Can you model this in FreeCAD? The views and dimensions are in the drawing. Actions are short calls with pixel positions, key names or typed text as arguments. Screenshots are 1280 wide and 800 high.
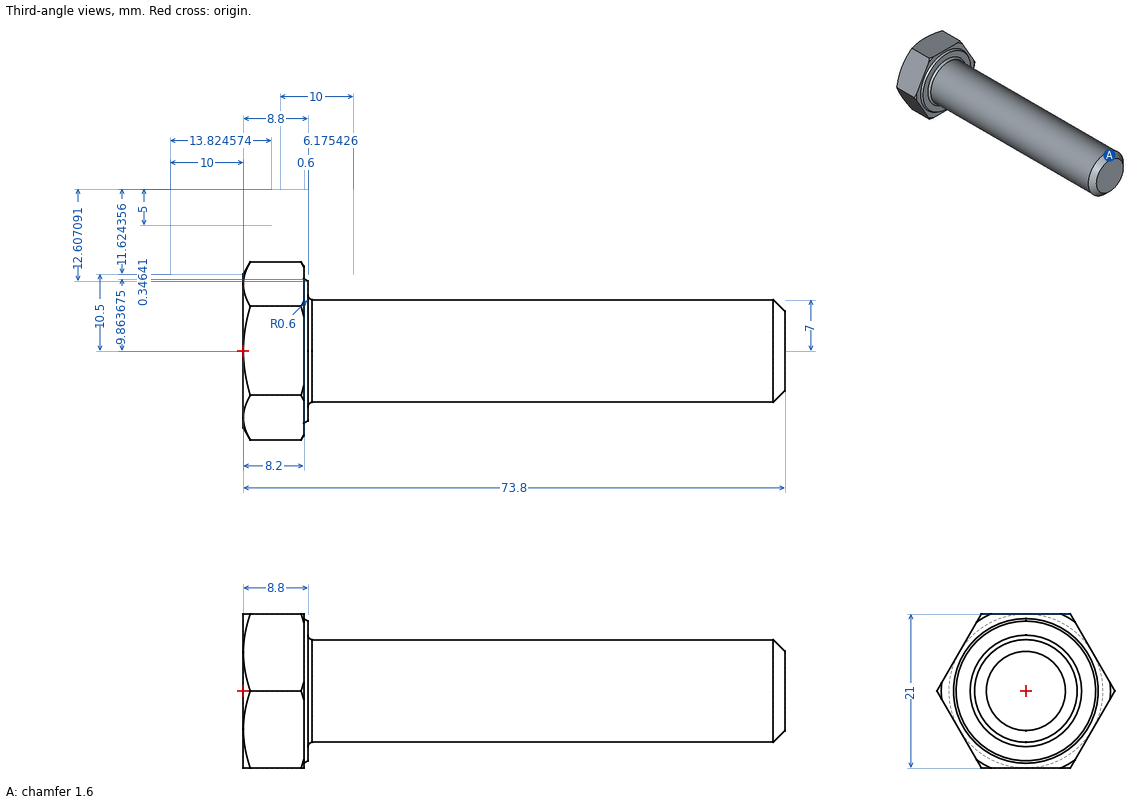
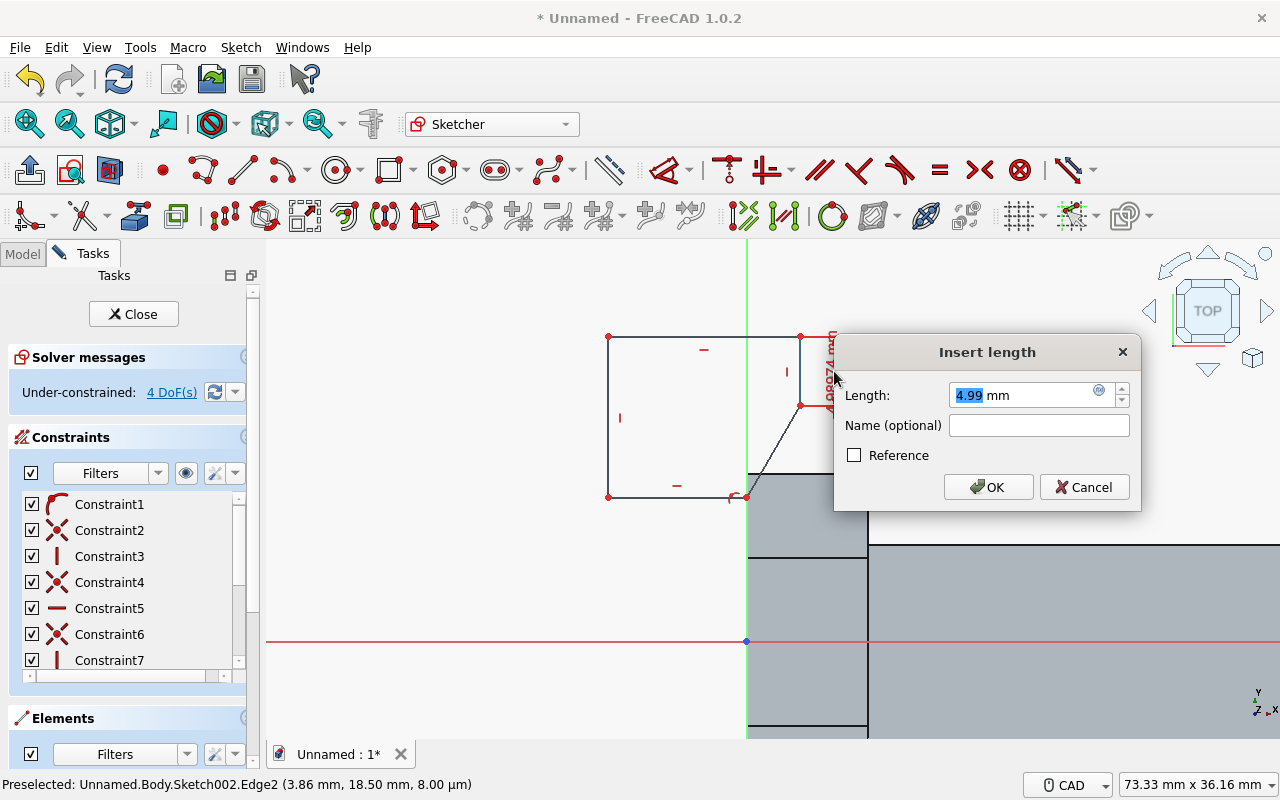
text(5)
key(Return)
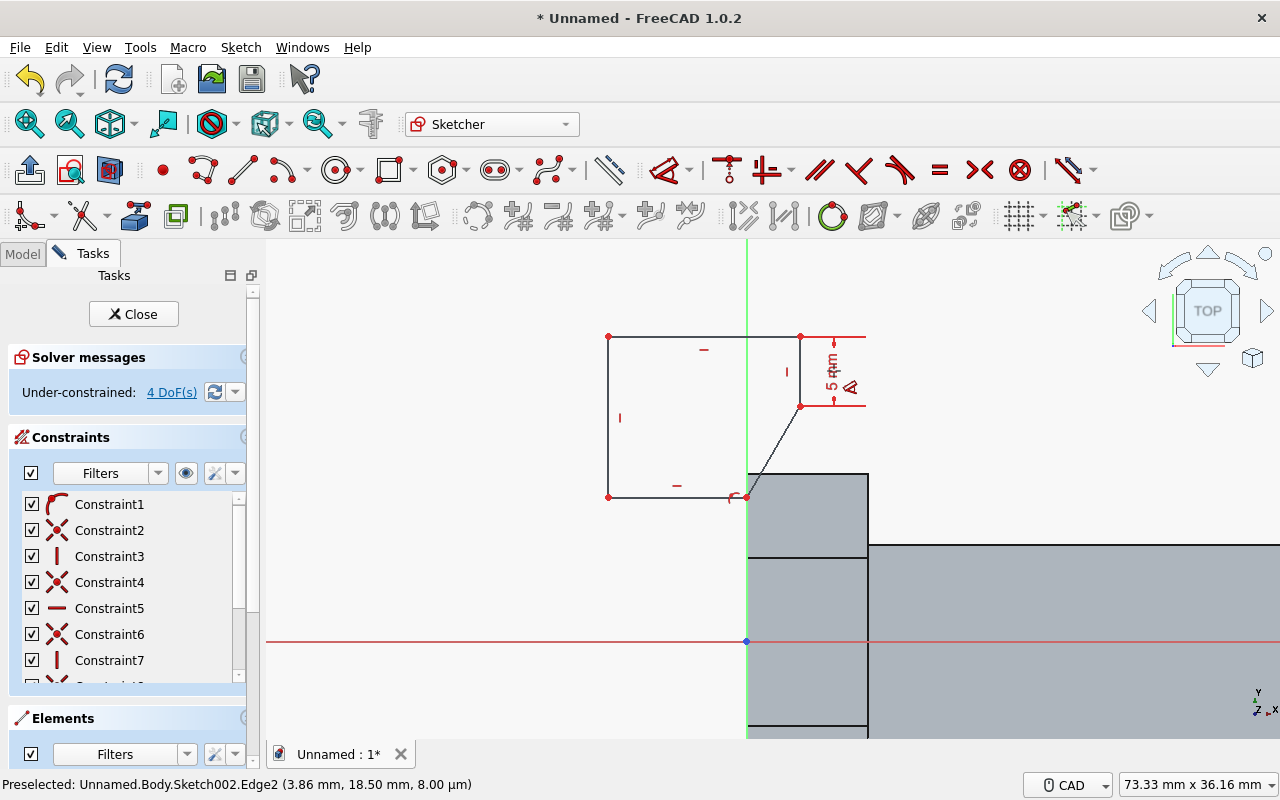
click(650, 498)
click(677, 532)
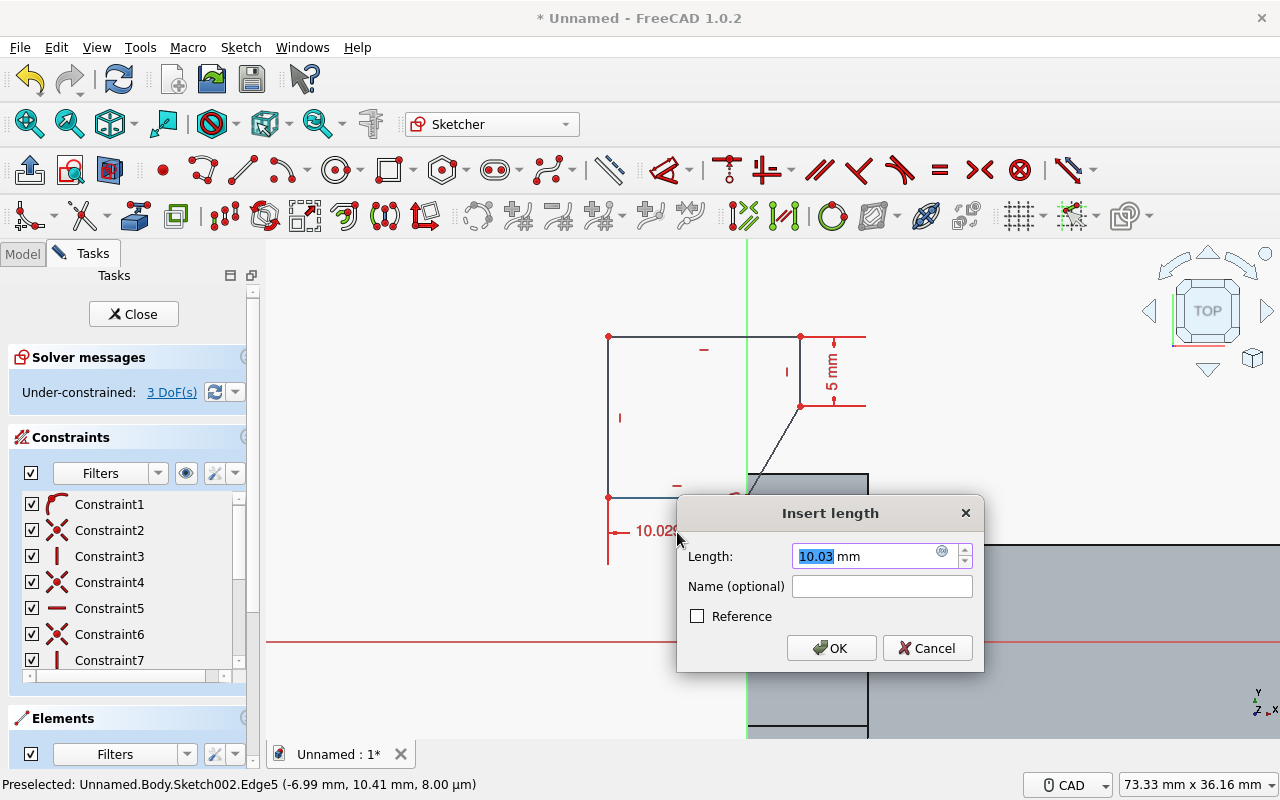
text(10)
key(Return)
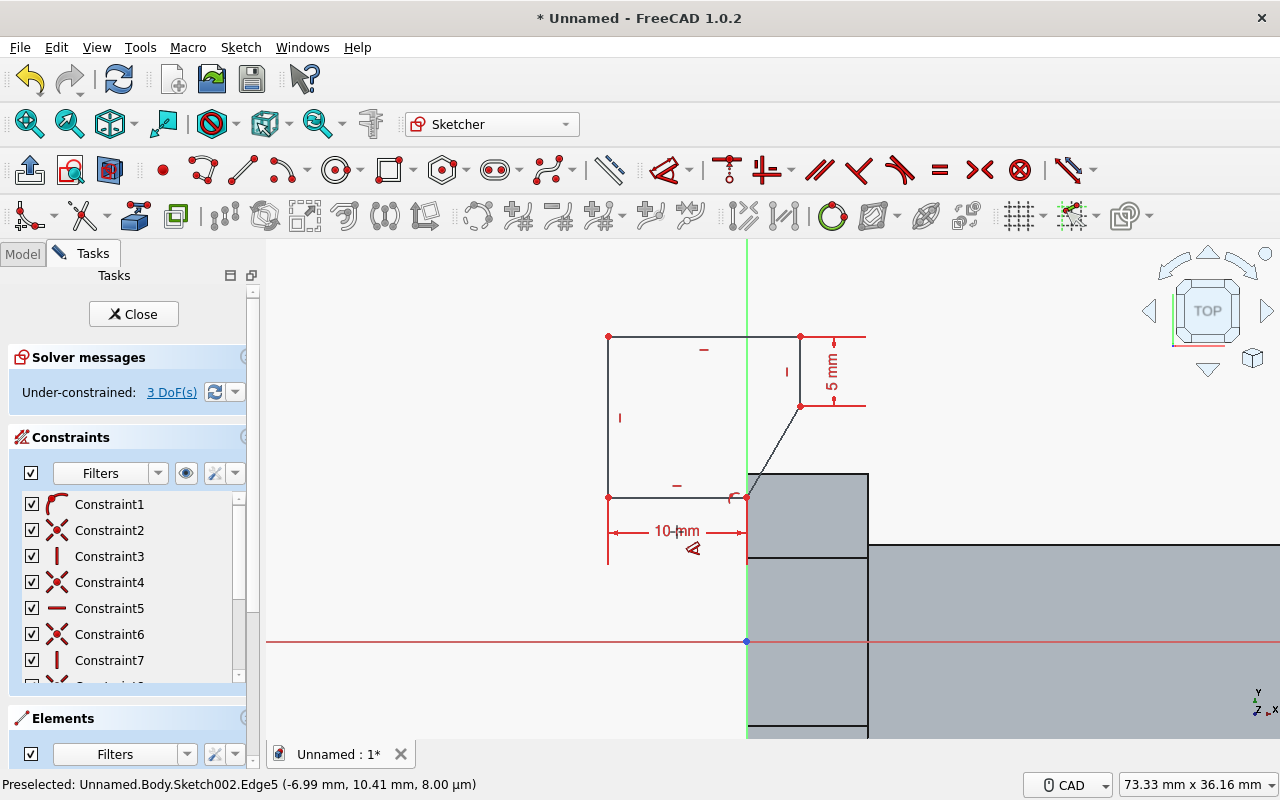
click(747, 498)
click(781, 570)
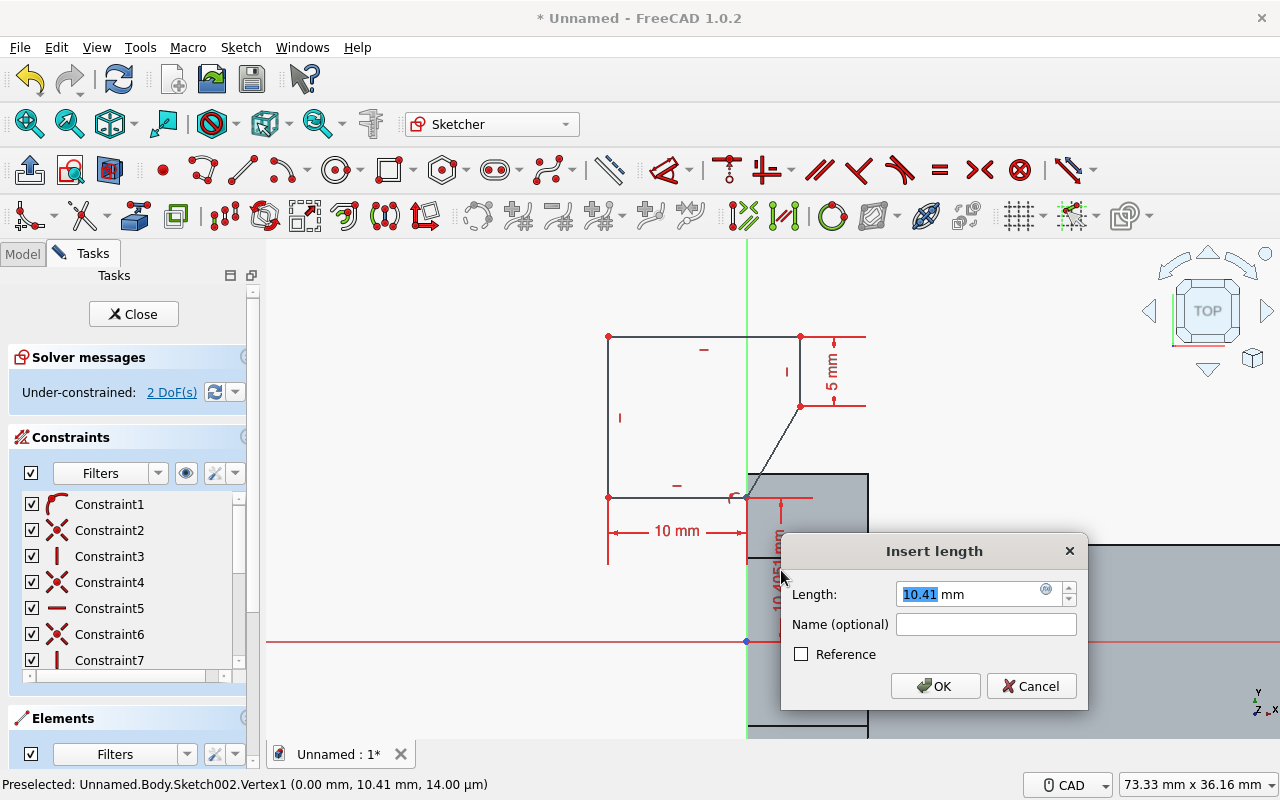
text(10.5)
key(Return)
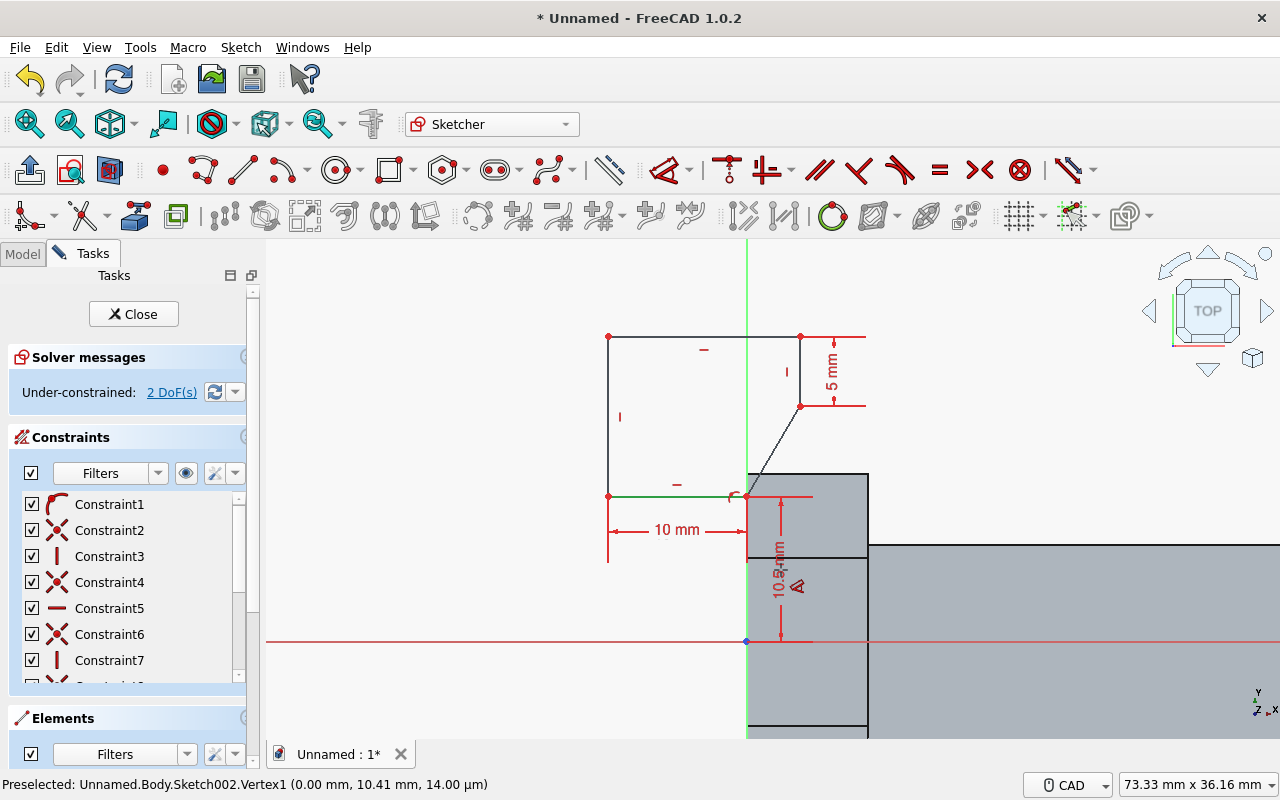
click(666, 337)
click(704, 303)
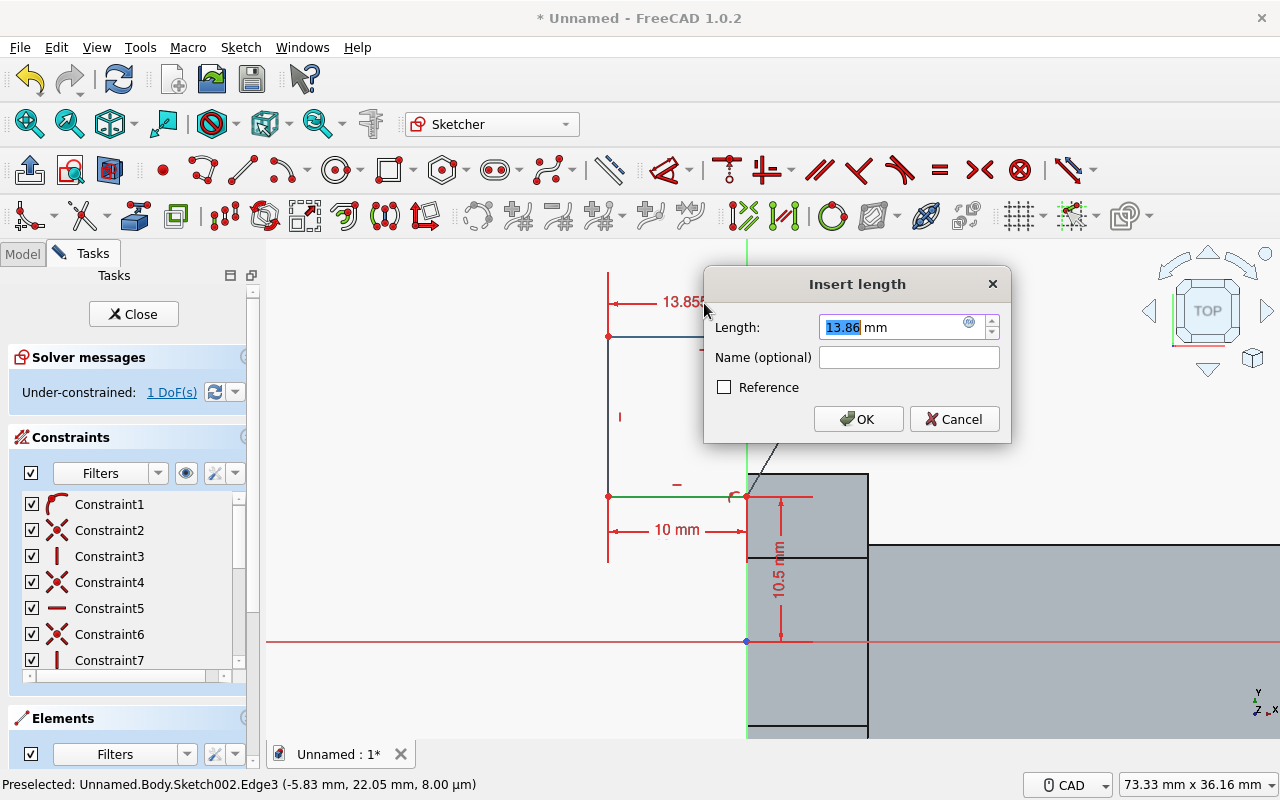
text(13.824574)
key(Return)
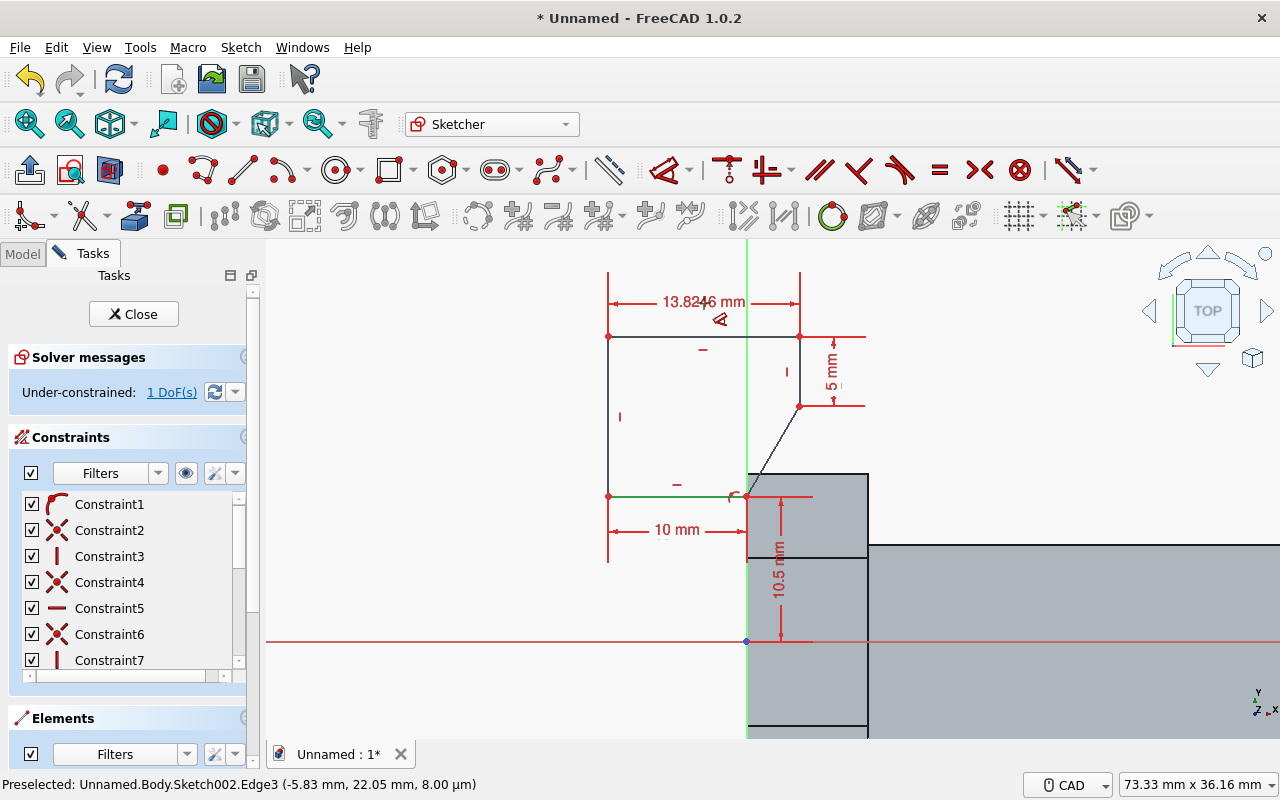
click(608, 385)
click(574, 417)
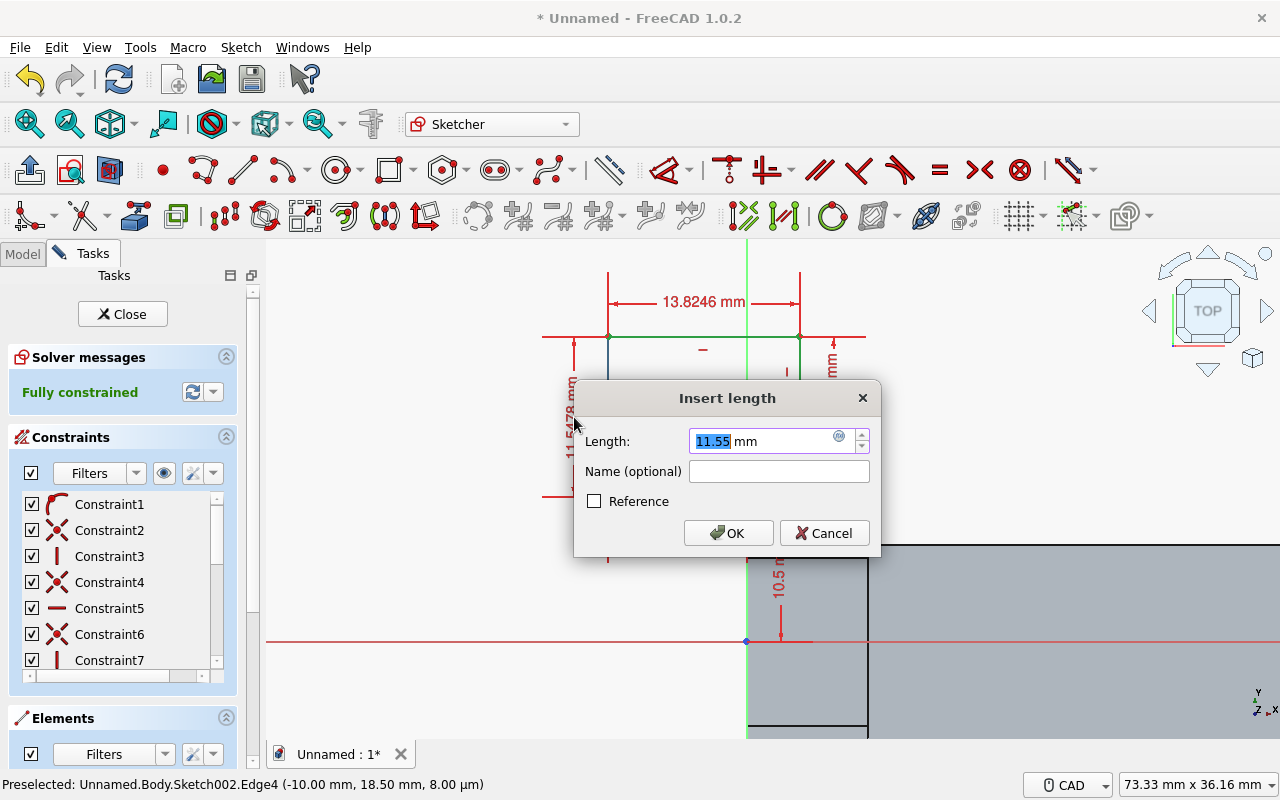
text(11.624356)
key(Return)
key(Escape)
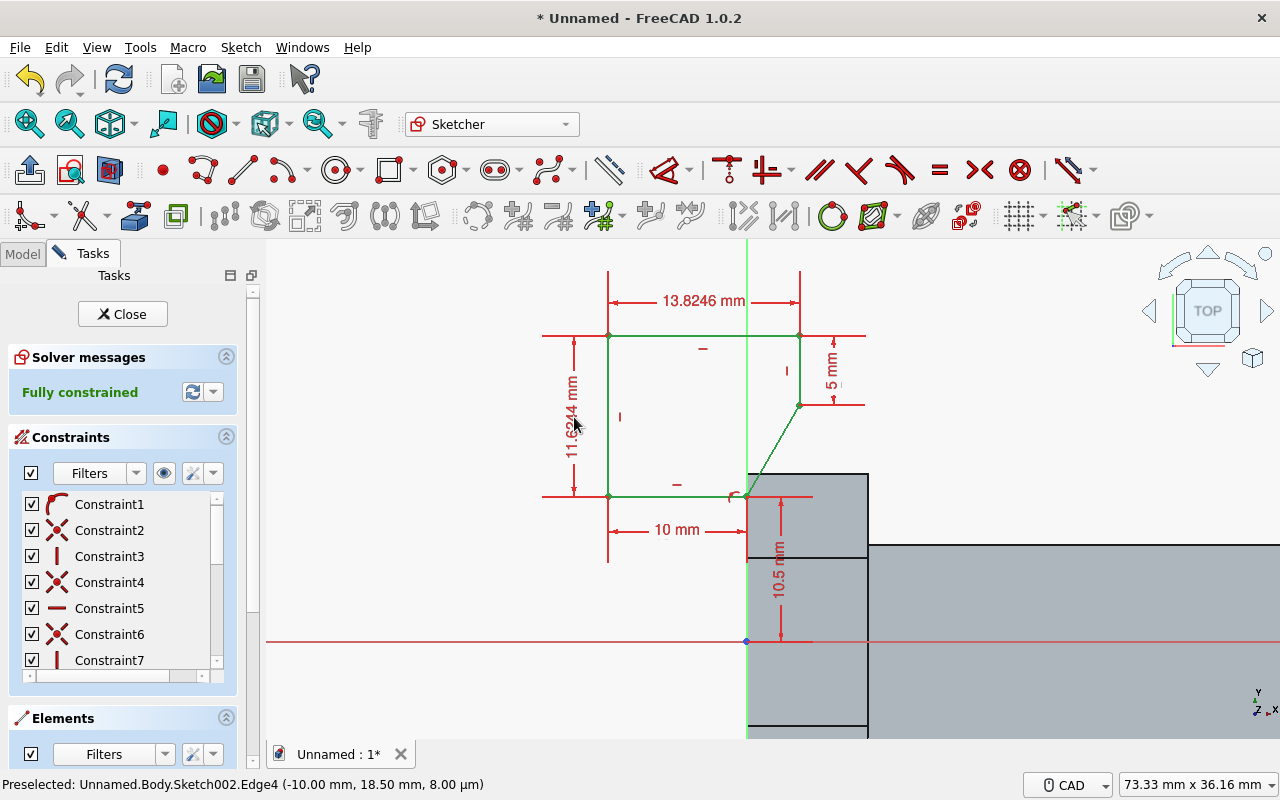
click(123, 314)